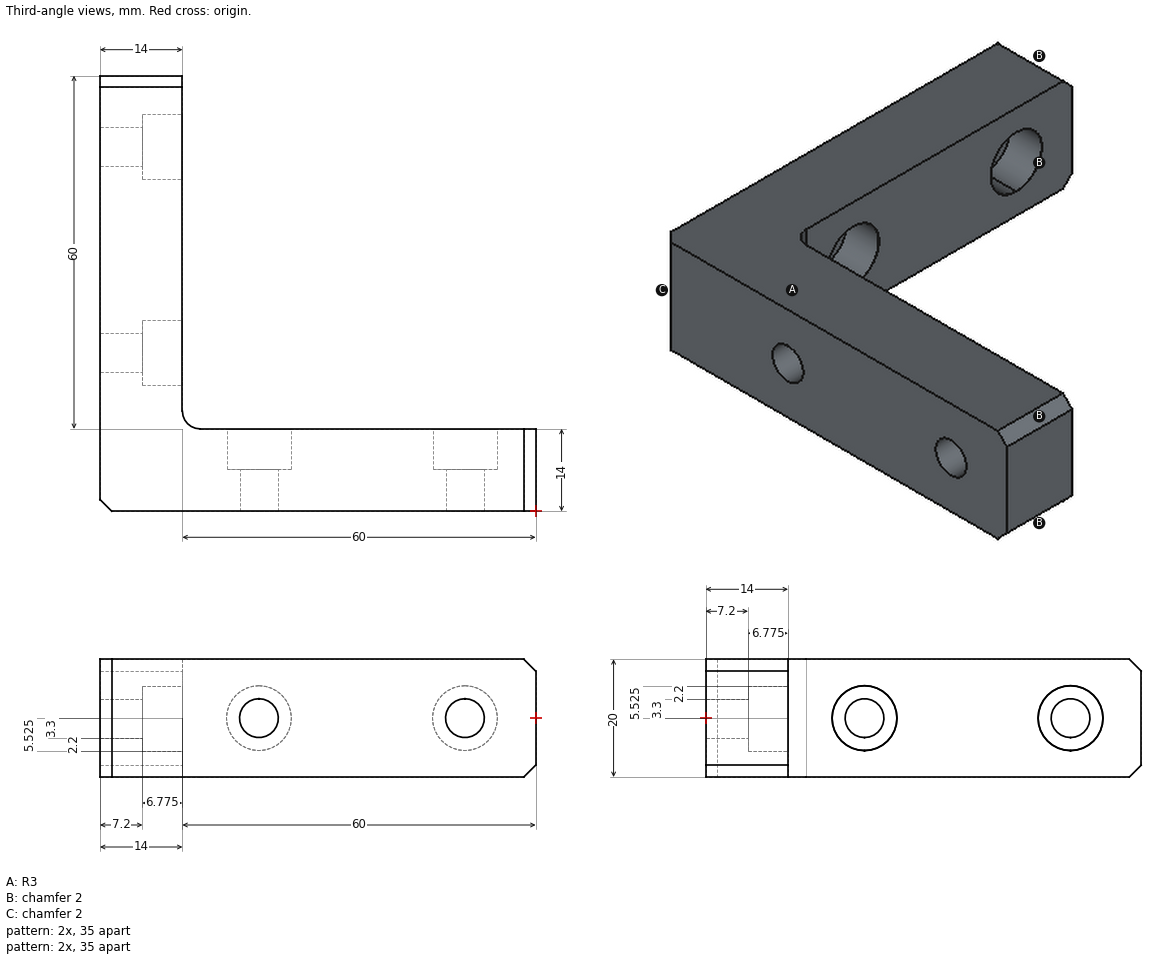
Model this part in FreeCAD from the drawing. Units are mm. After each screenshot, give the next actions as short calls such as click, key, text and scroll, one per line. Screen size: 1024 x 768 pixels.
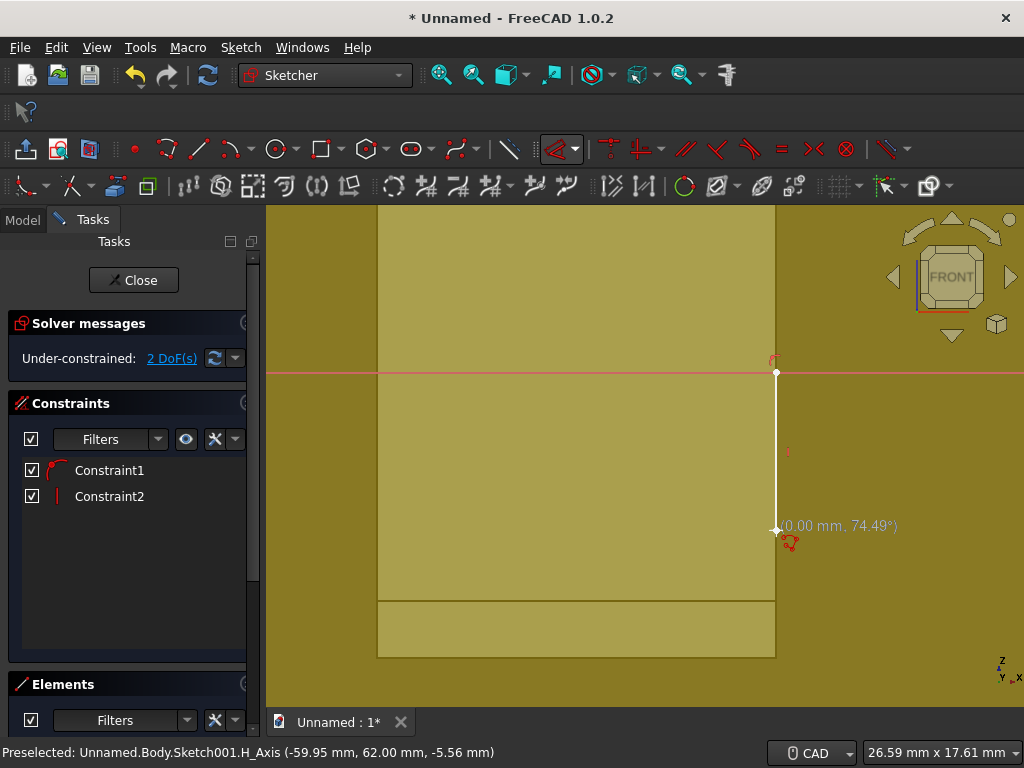
scroll(775, 529, up, 16)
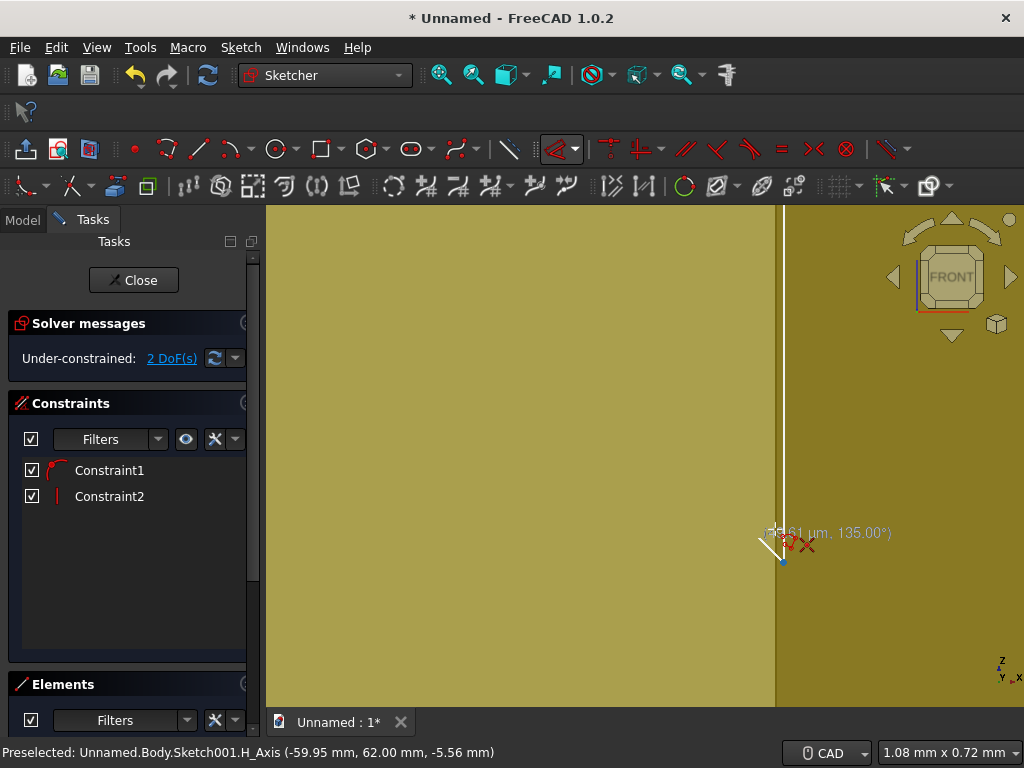
click(758, 521)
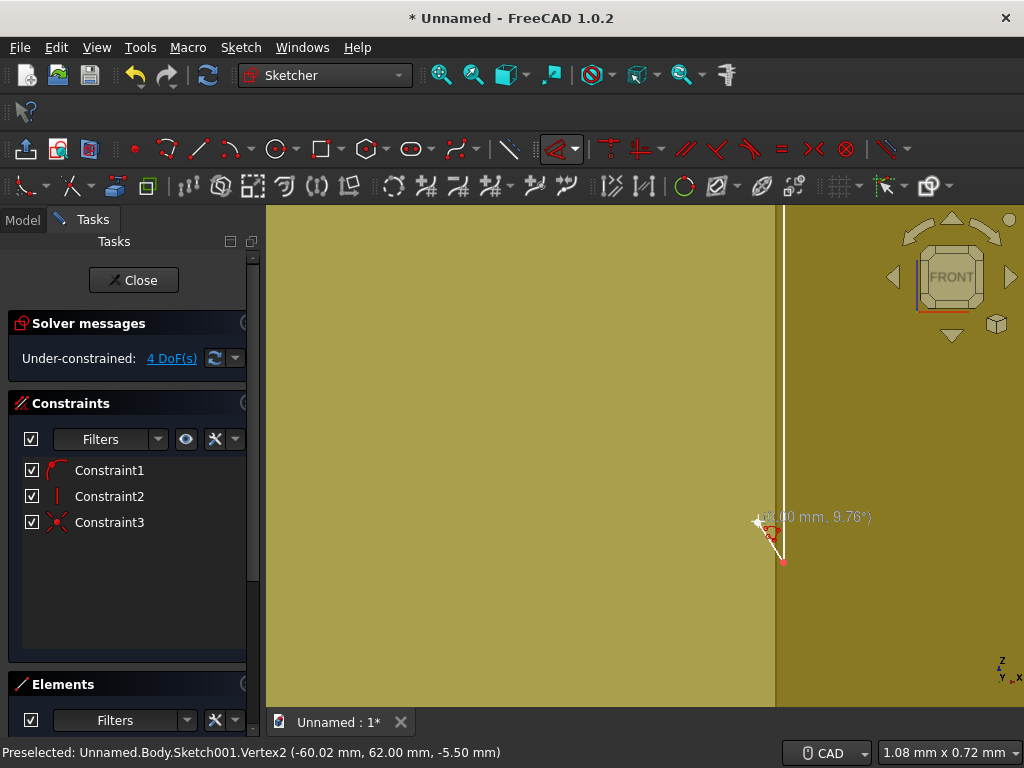
scroll(823, 553, down, 15)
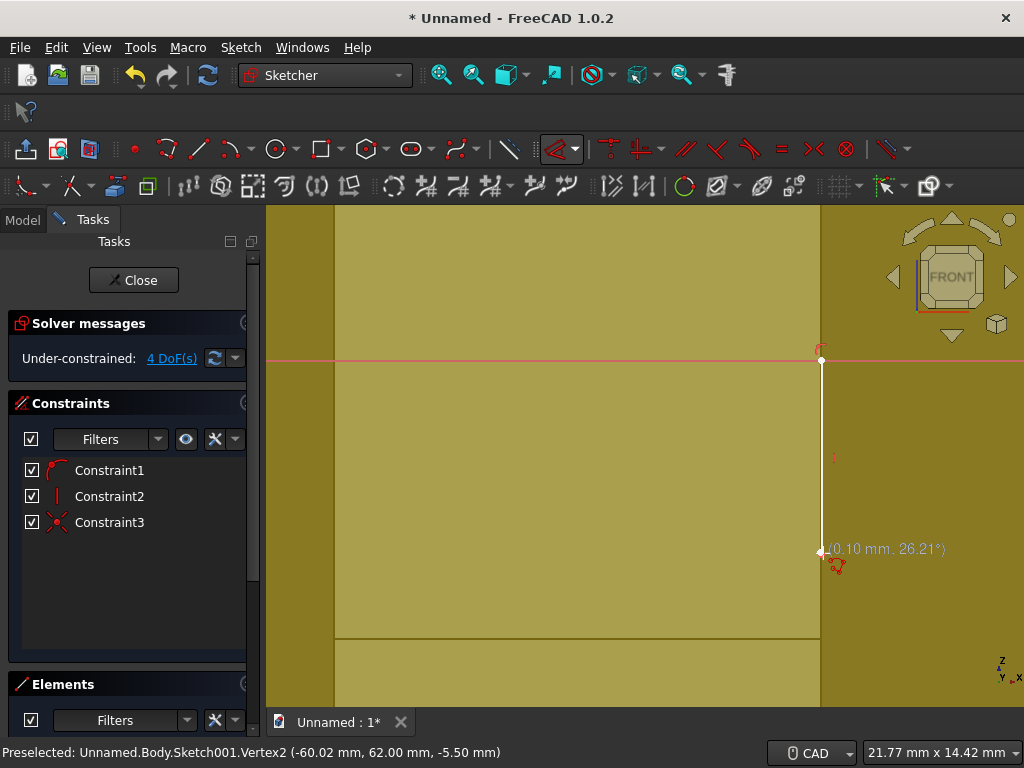
click(585, 552)
click(585, 475)
click(334, 475)
click(334, 370)
click(822, 361)
key(Escape)
key(Escape)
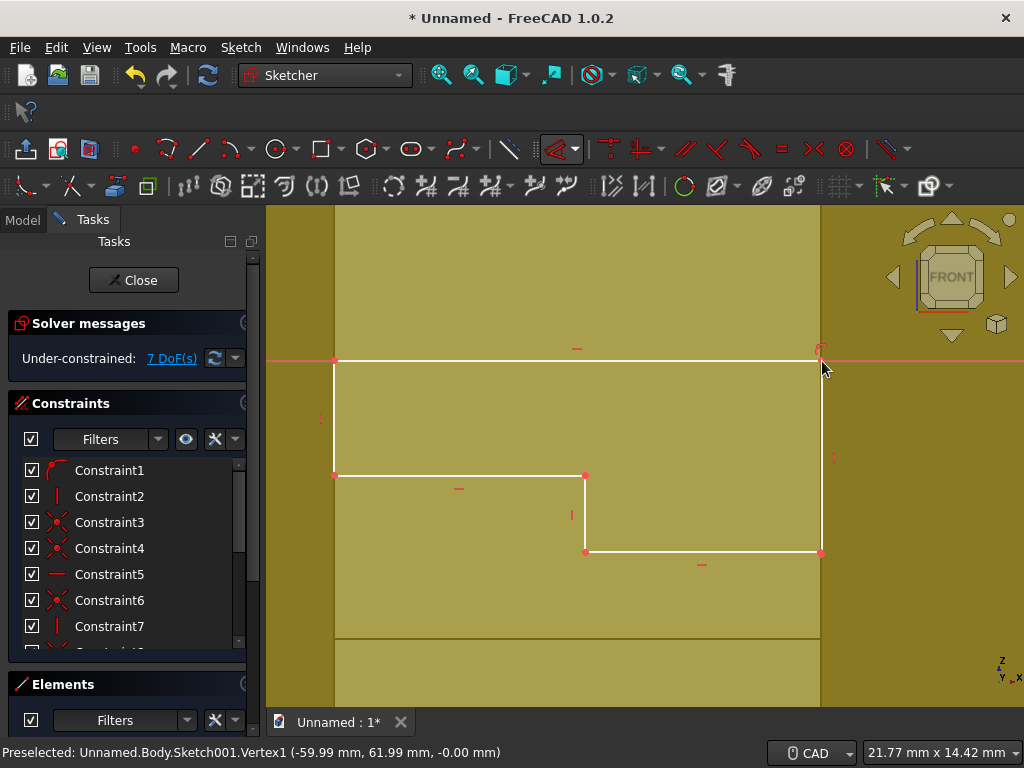
click(480, 361)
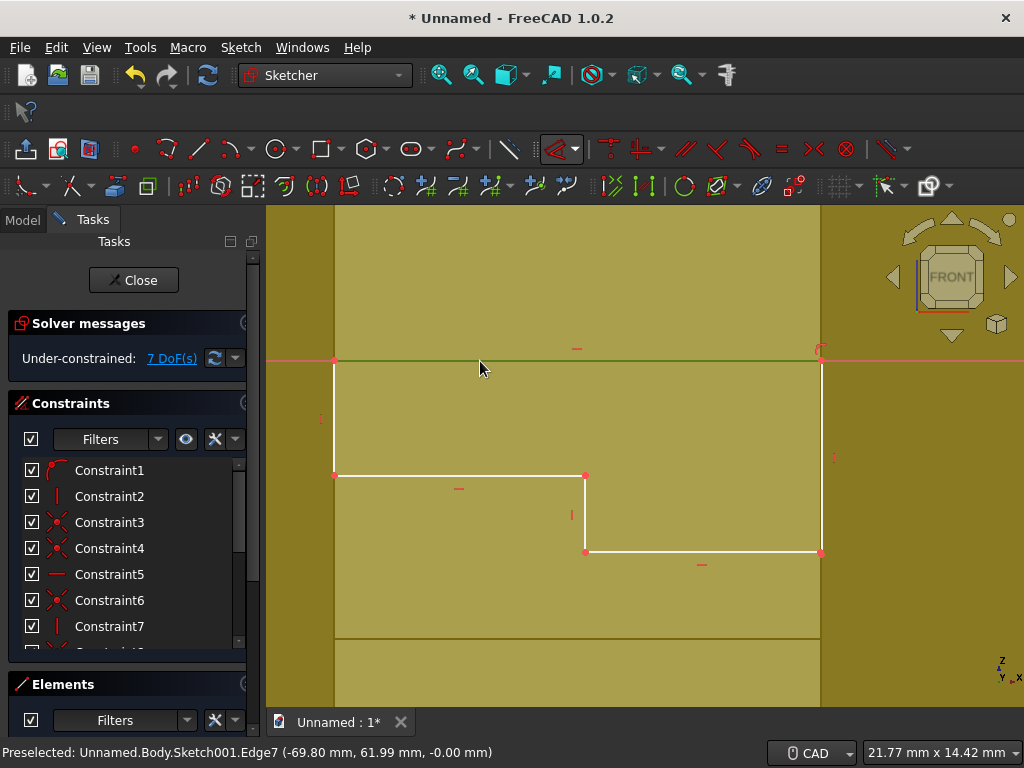
click(578, 150)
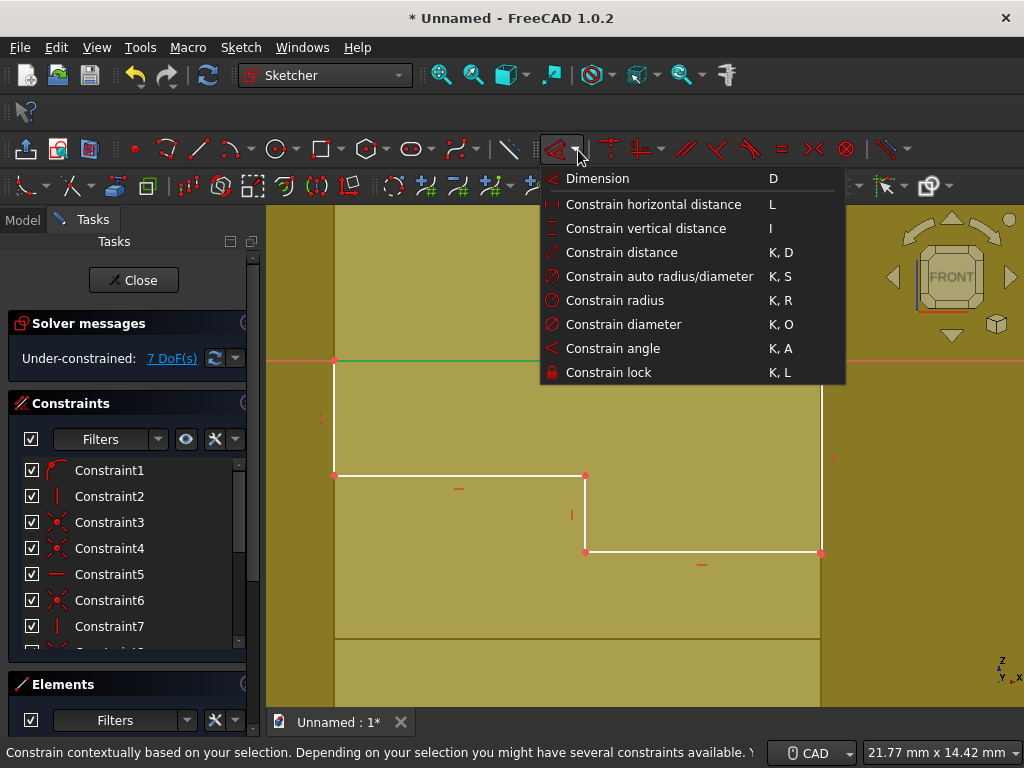
click(693, 204)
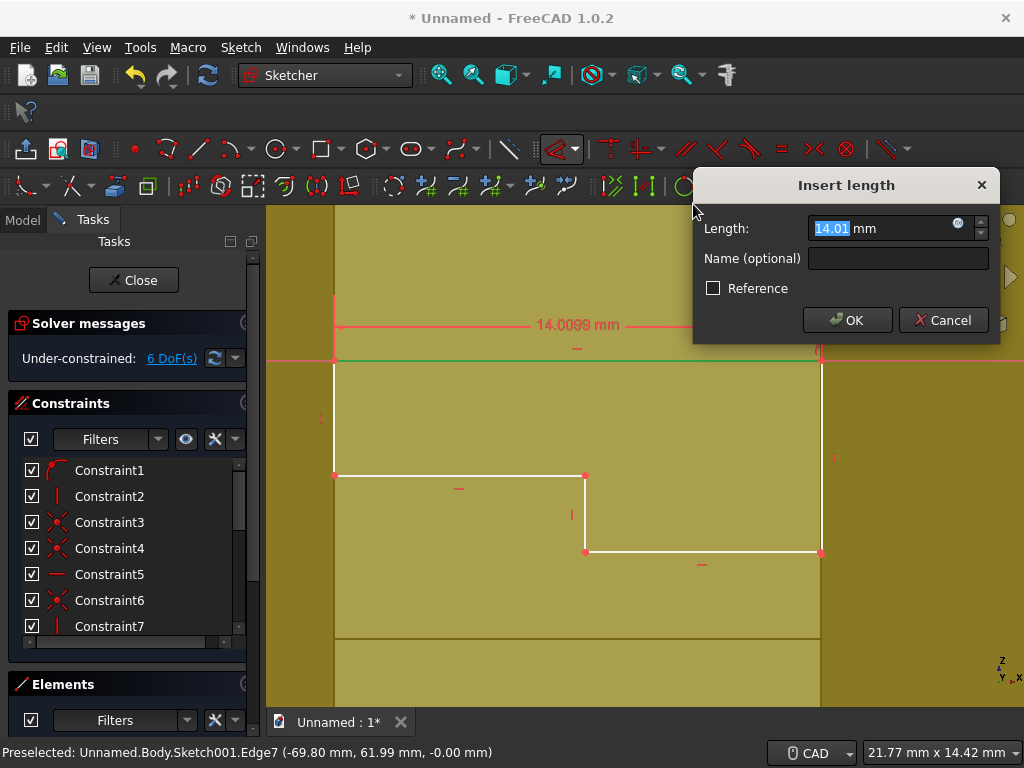
text(14)
key(Return)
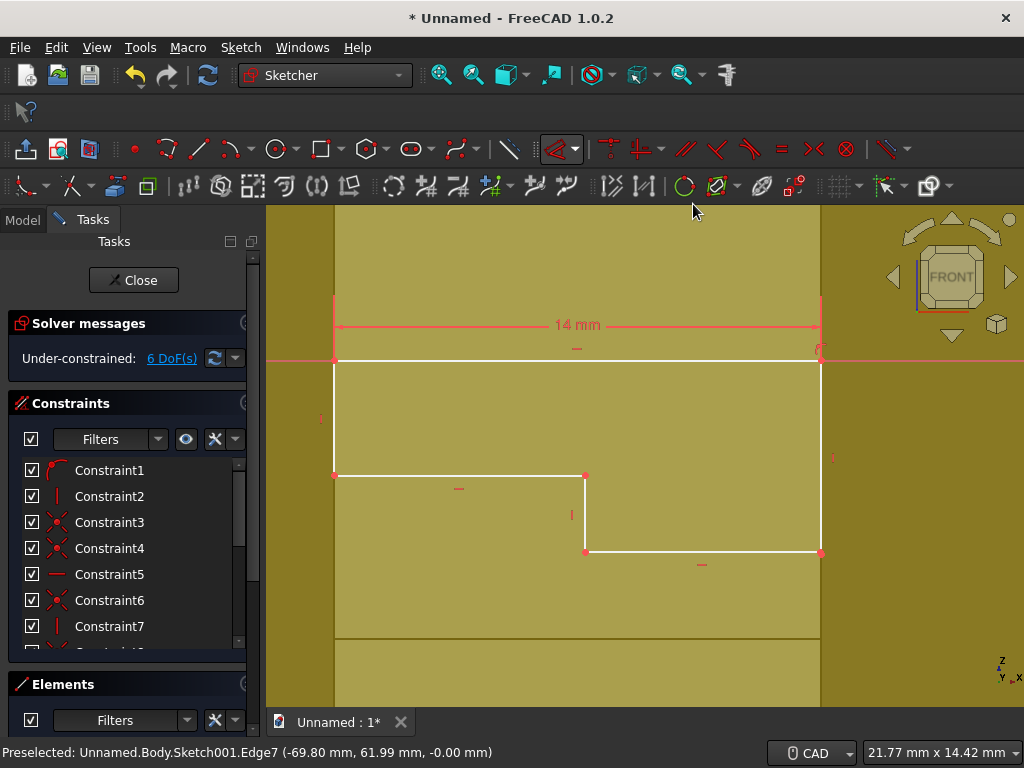
click(585, 529)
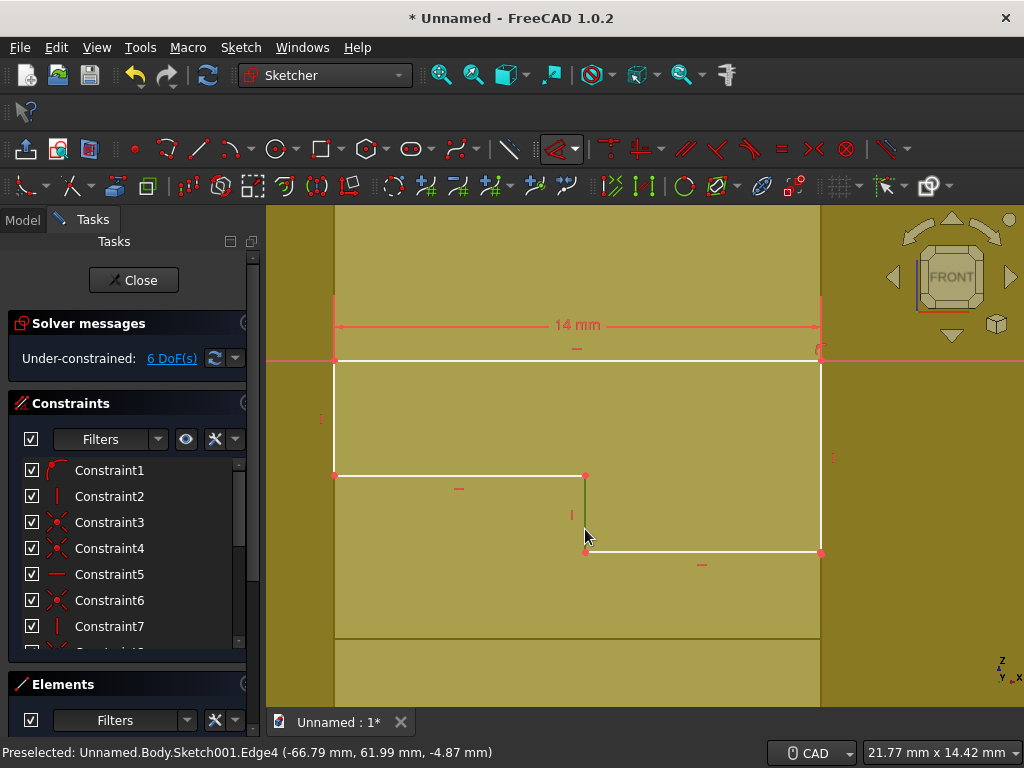
key(i)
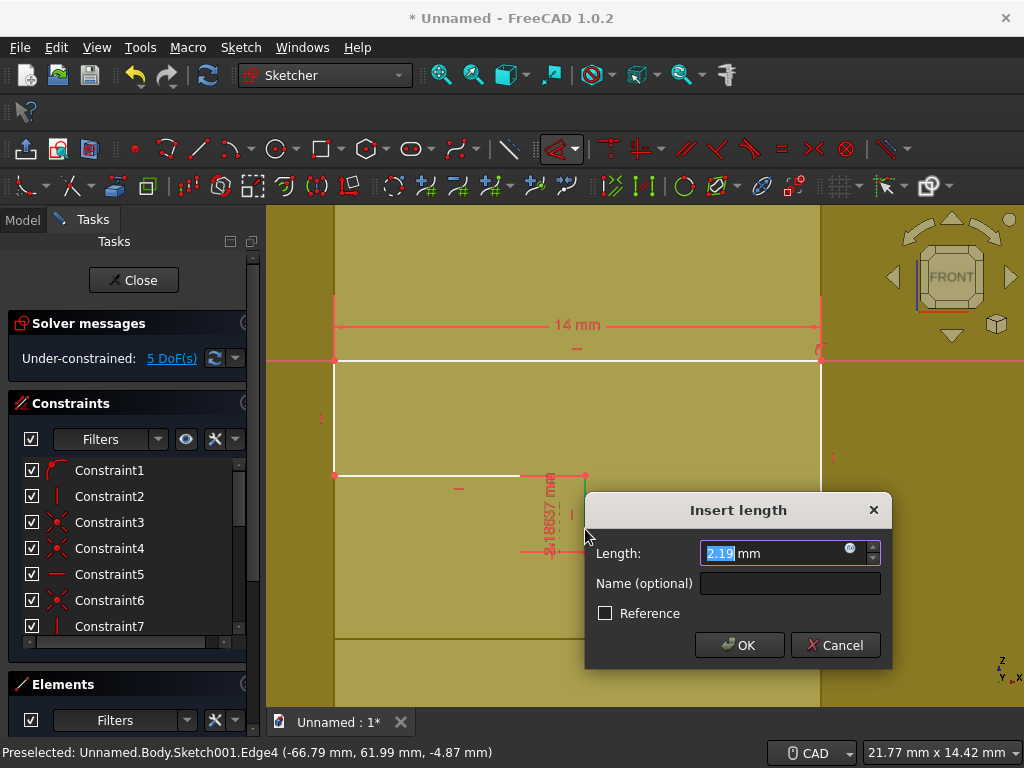
text(2.2)
key(Return)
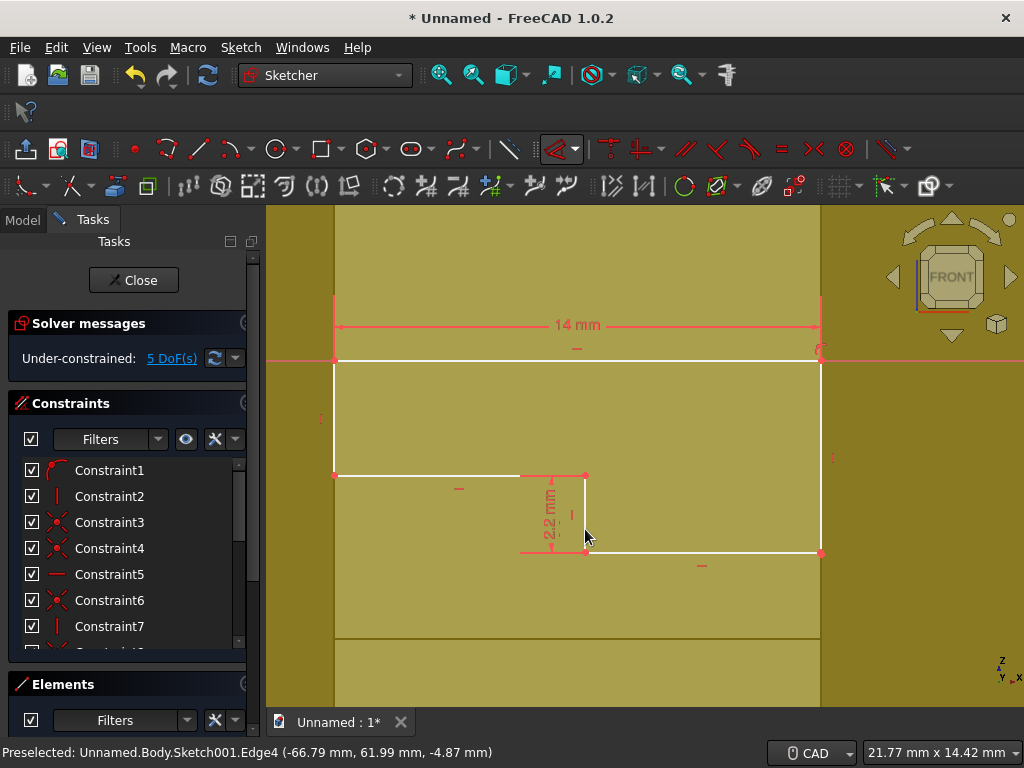
click(510, 476)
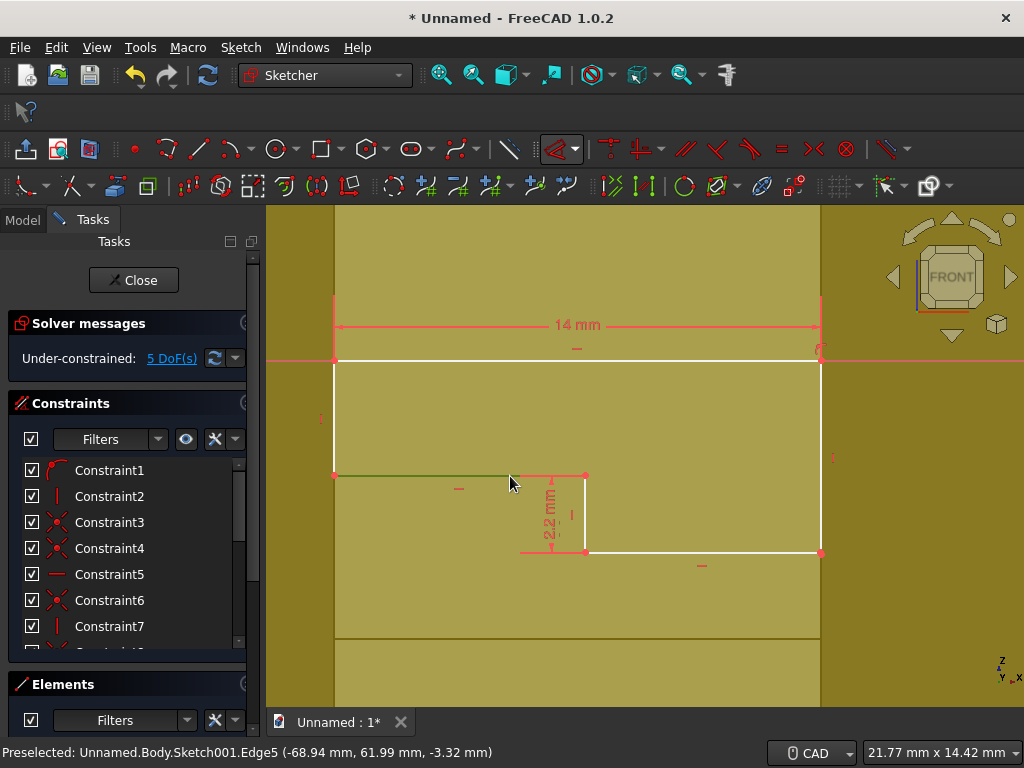
key(l)